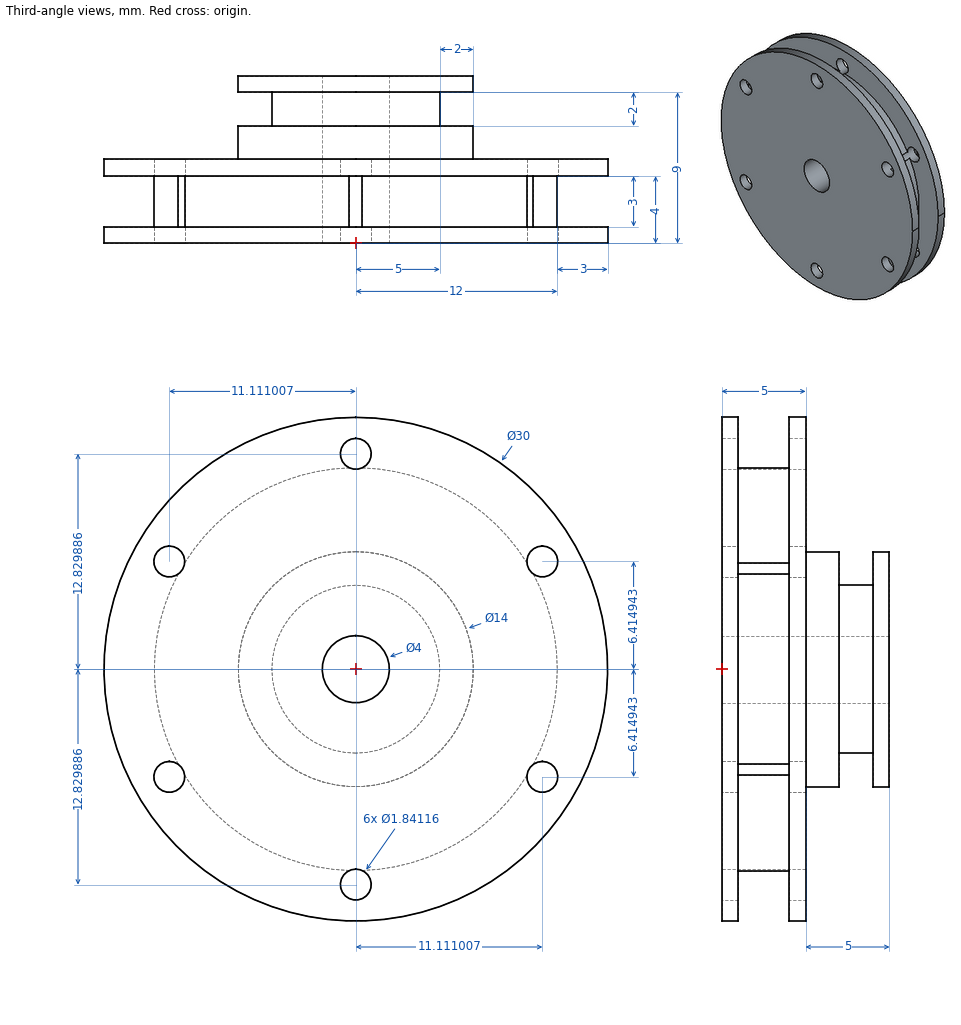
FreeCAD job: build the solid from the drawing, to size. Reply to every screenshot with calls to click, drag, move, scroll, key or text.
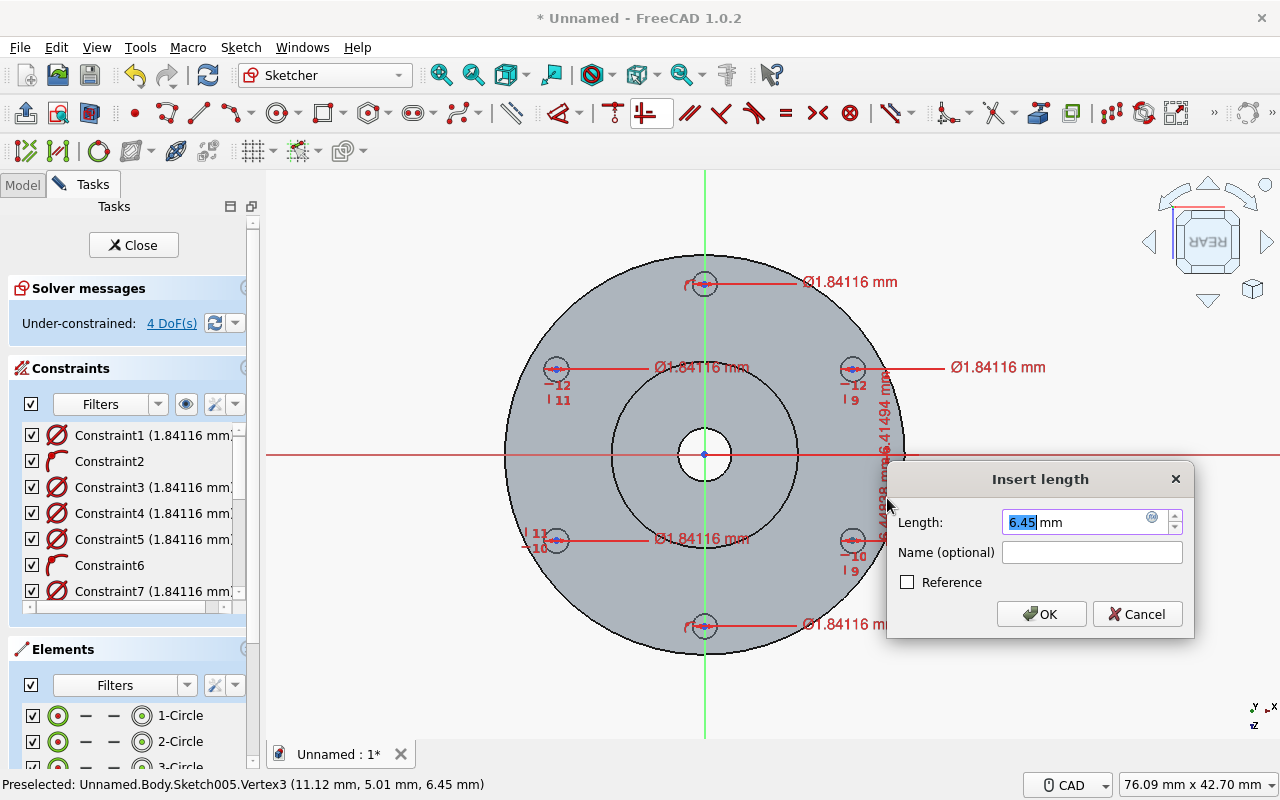
text(6.414943)
key(Return)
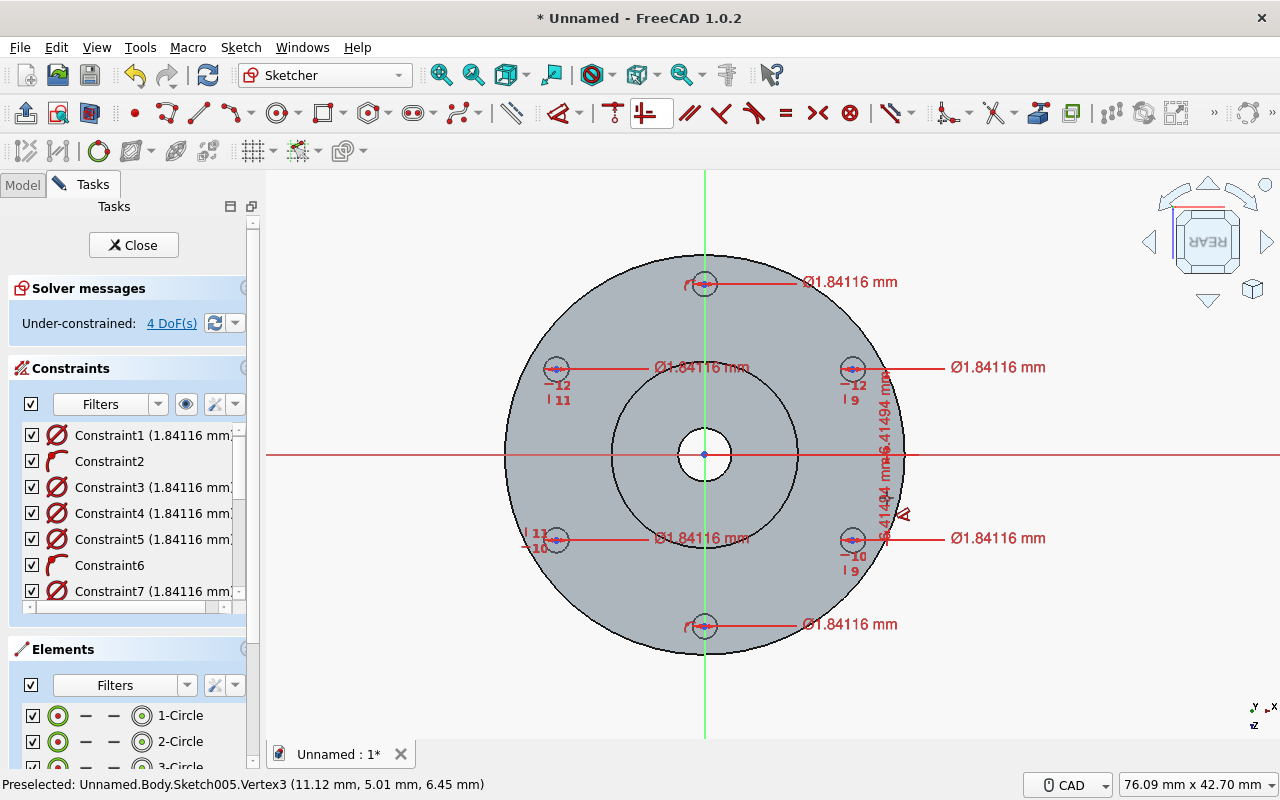
click(705, 284)
click(739, 370)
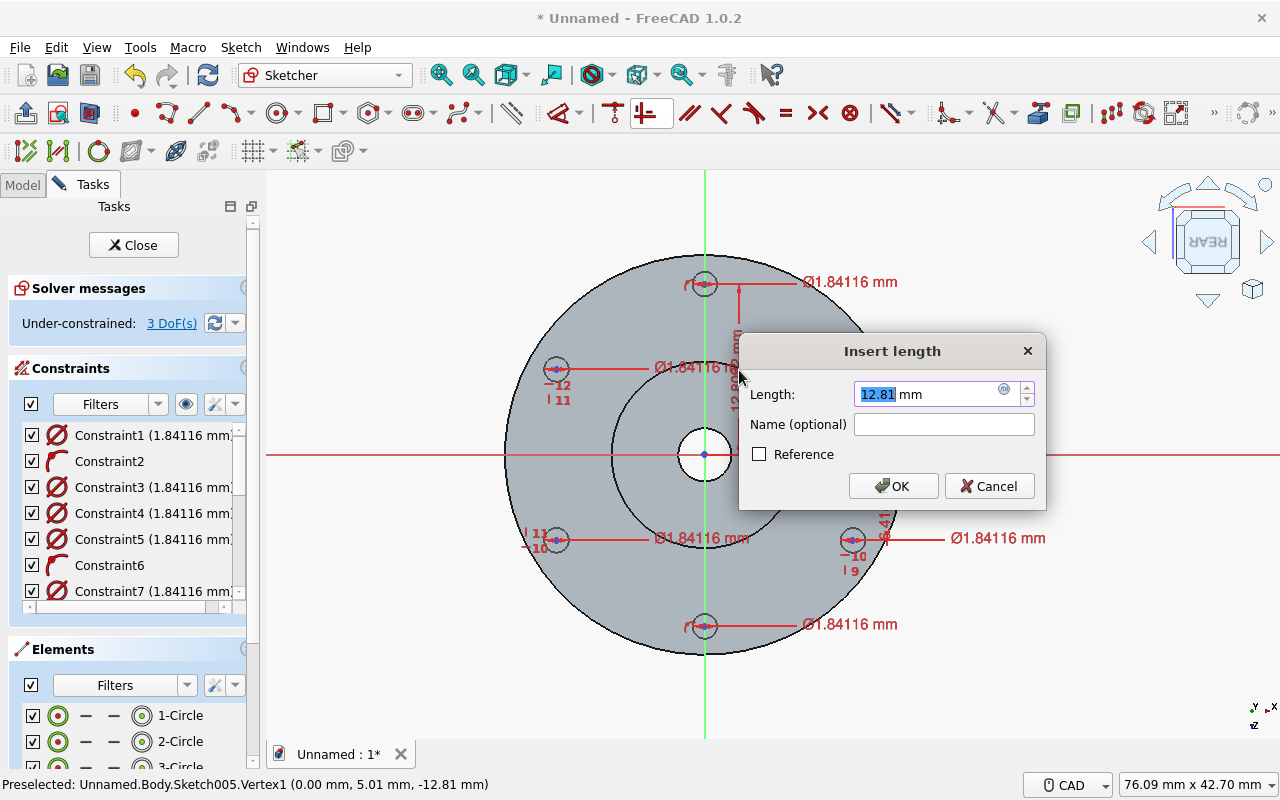
text(12.829886)
key(Return)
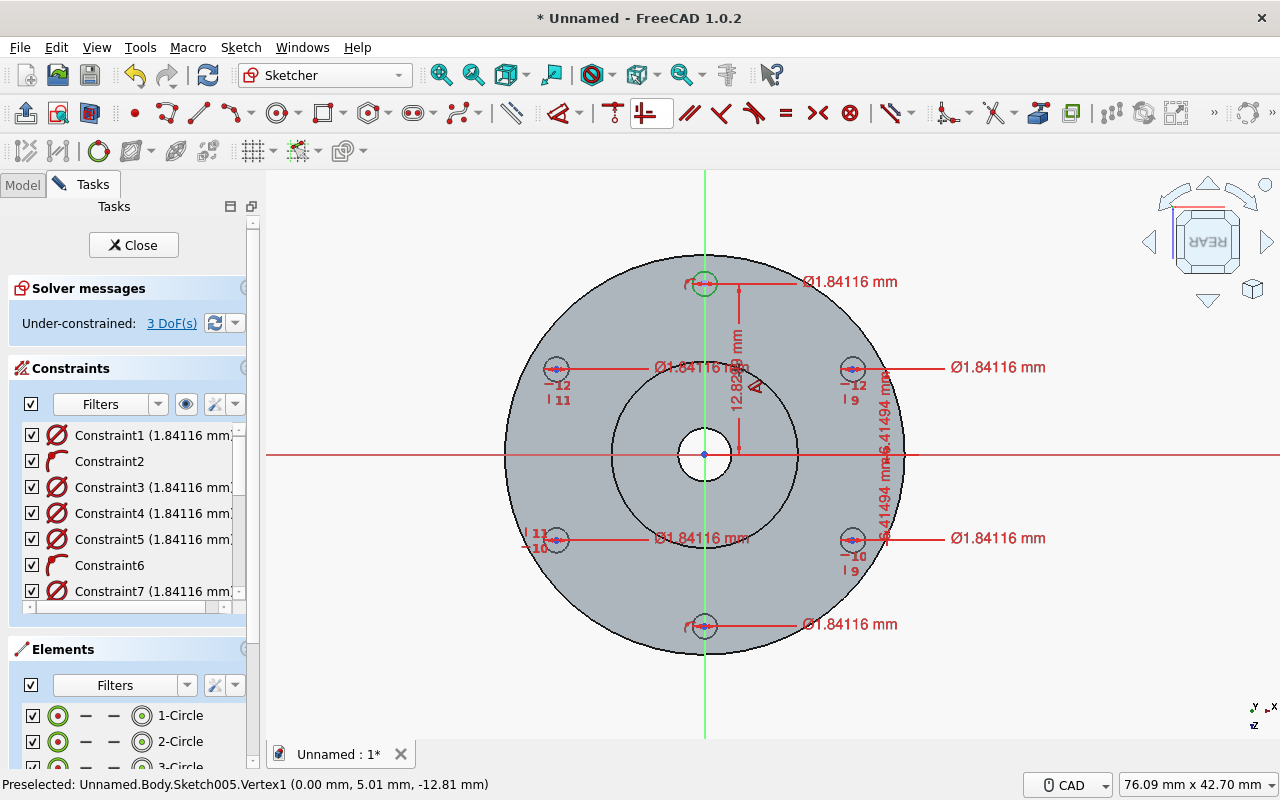
click(853, 369)
click(779, 335)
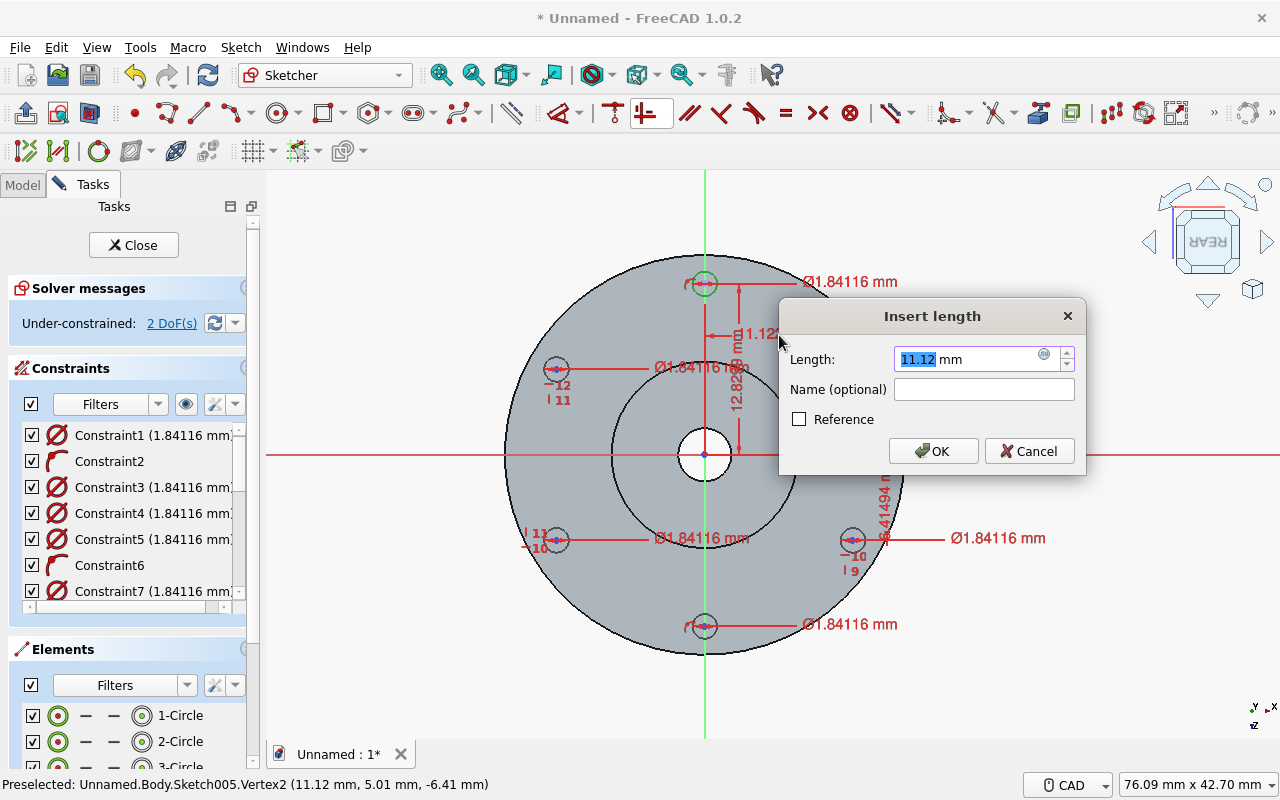
text(11.111007)
key(Return)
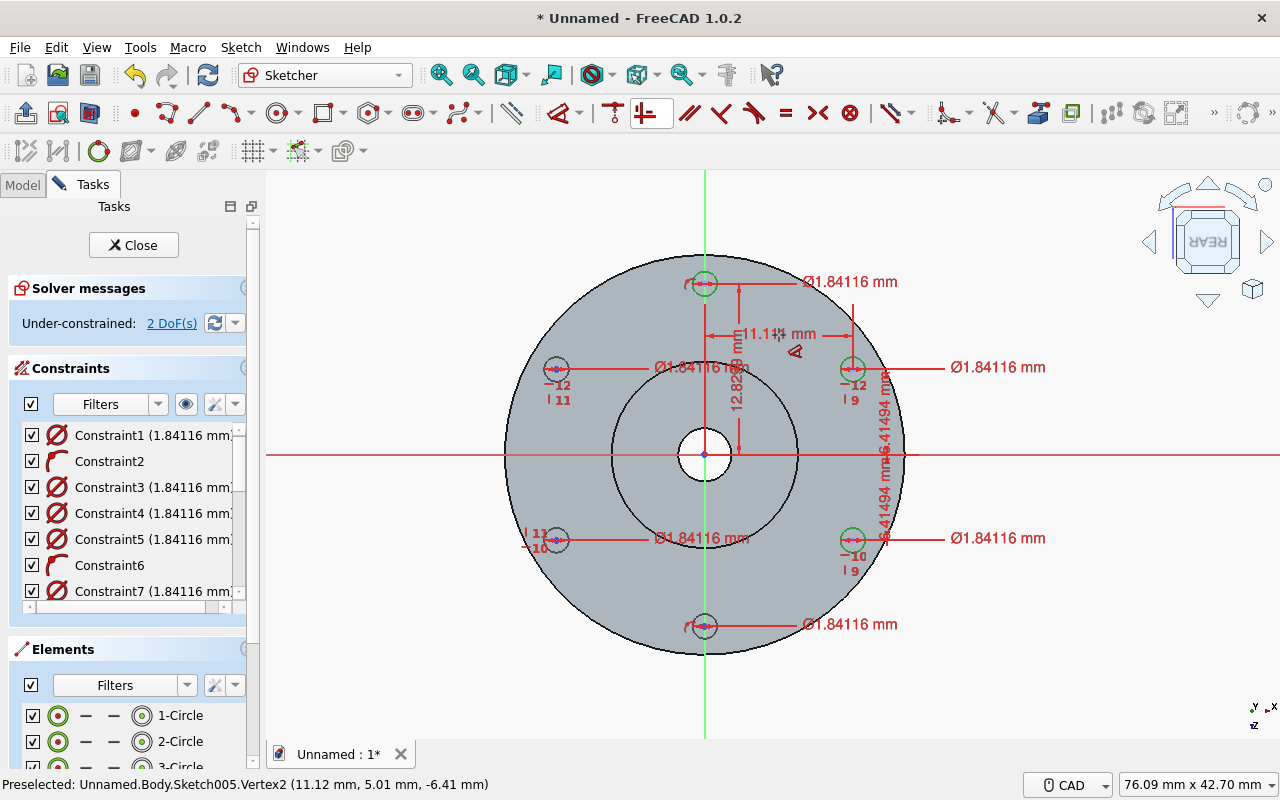
click(705, 626)
click(739, 541)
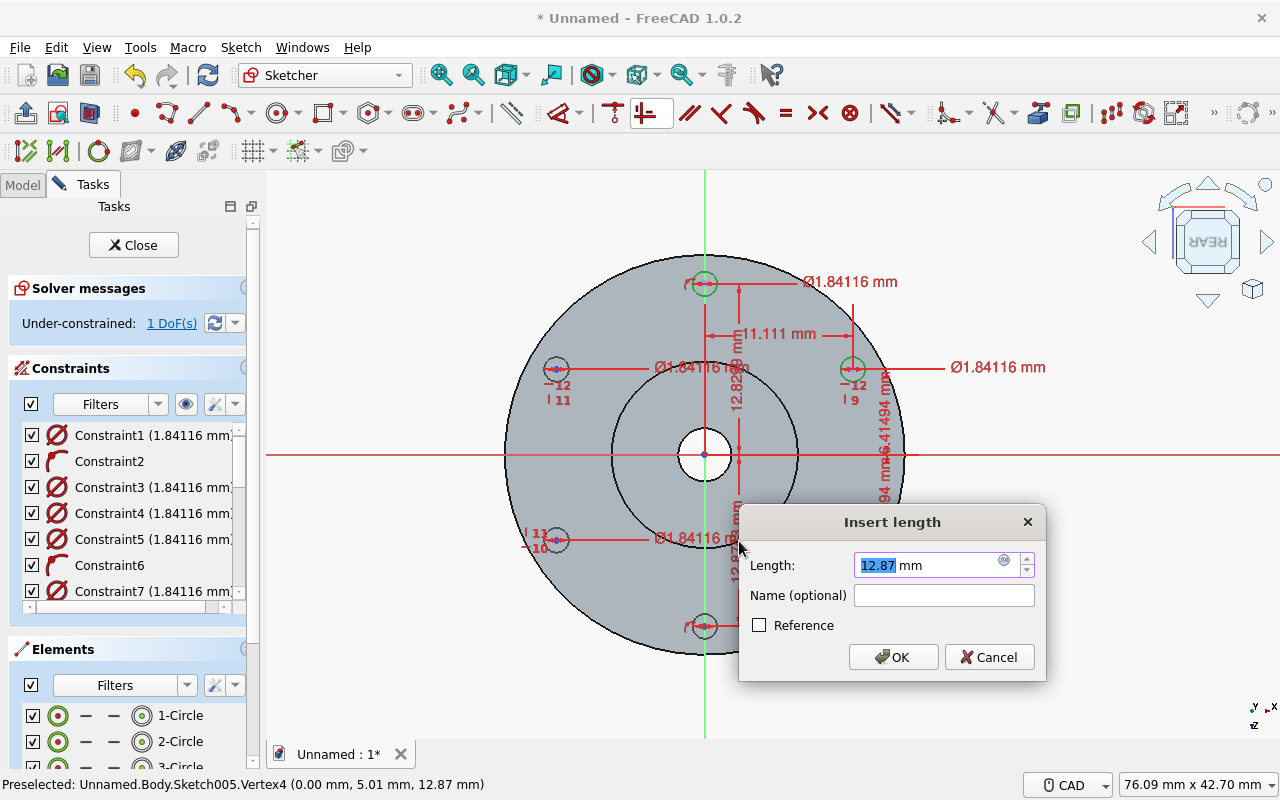
text(12.829886)
key(Return)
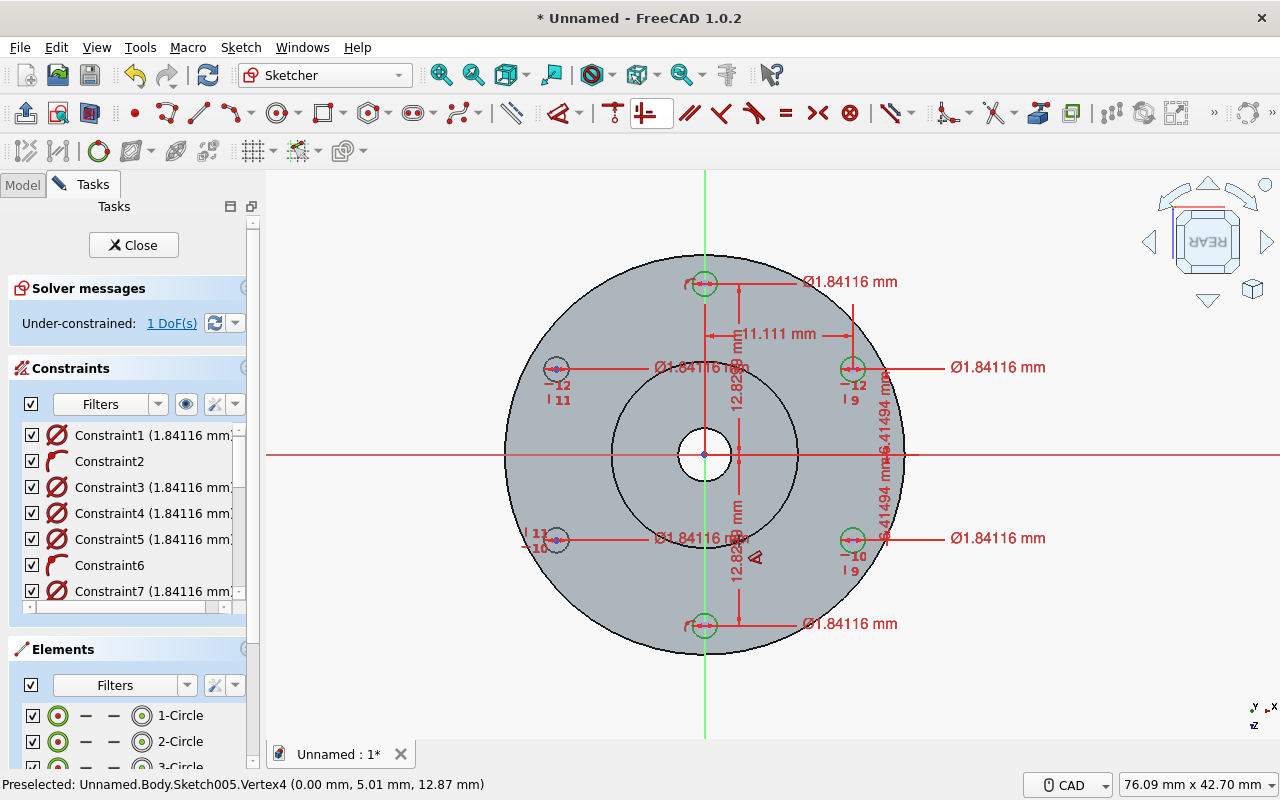
click(557, 540)
click(631, 574)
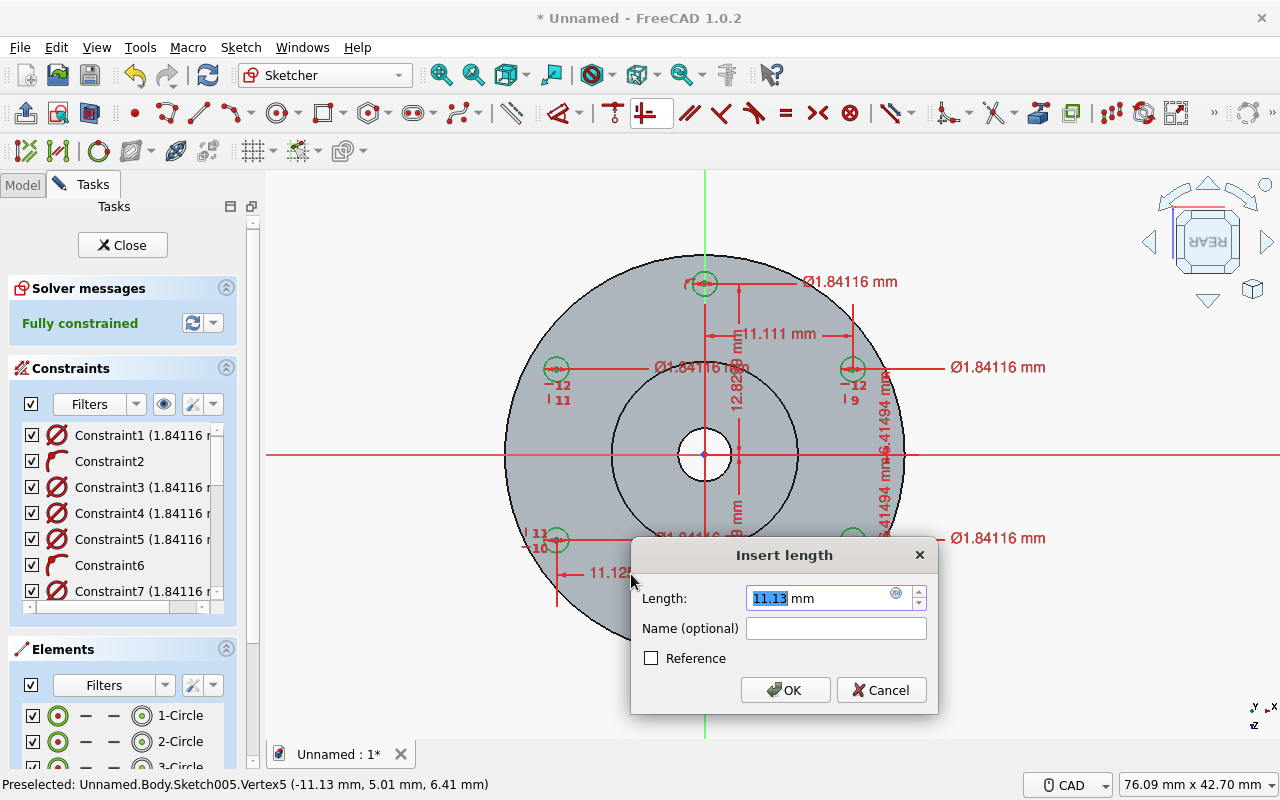
text(11.111007)
key(Return)
key(Escape)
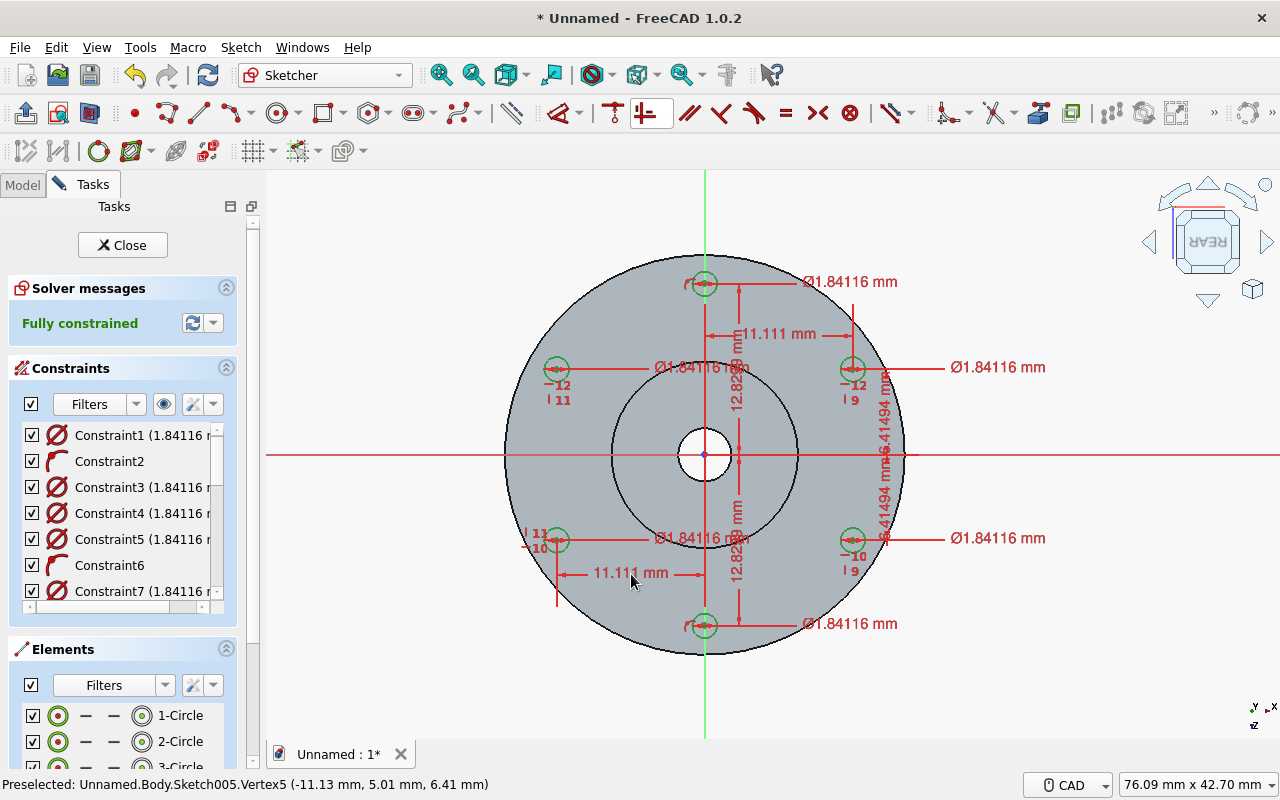
click(123, 245)